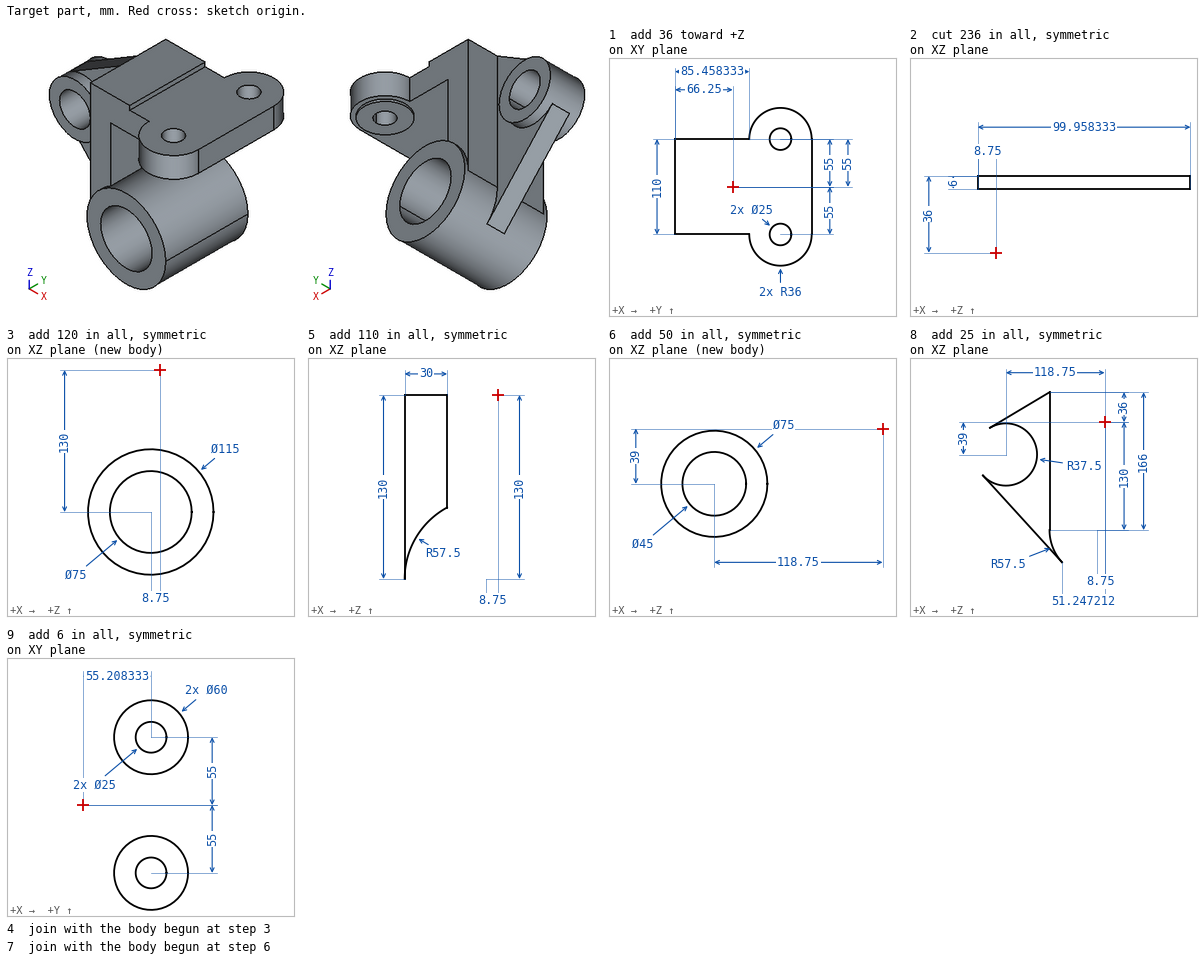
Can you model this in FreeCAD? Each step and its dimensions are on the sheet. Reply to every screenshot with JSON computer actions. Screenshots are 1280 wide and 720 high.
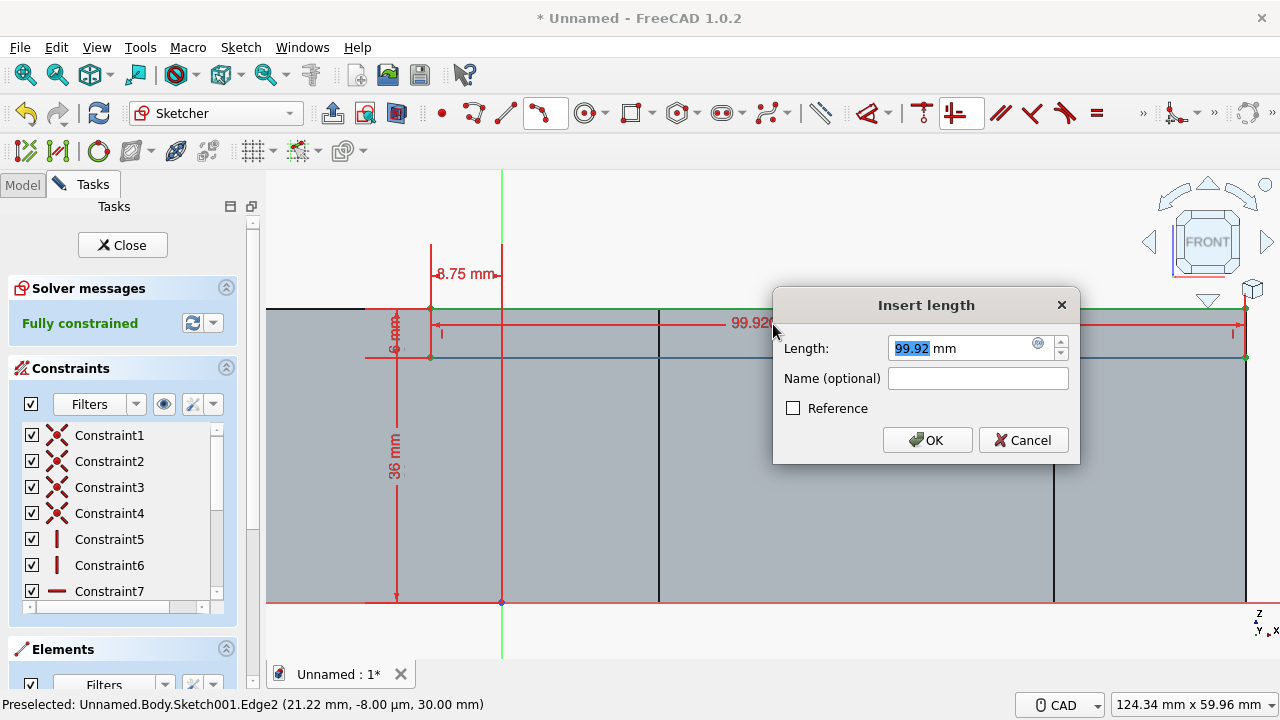
{"action": "type", "text": "99.958333"}
{"action": "key", "text": "Return"}
{"action": "key", "text": "Escape"}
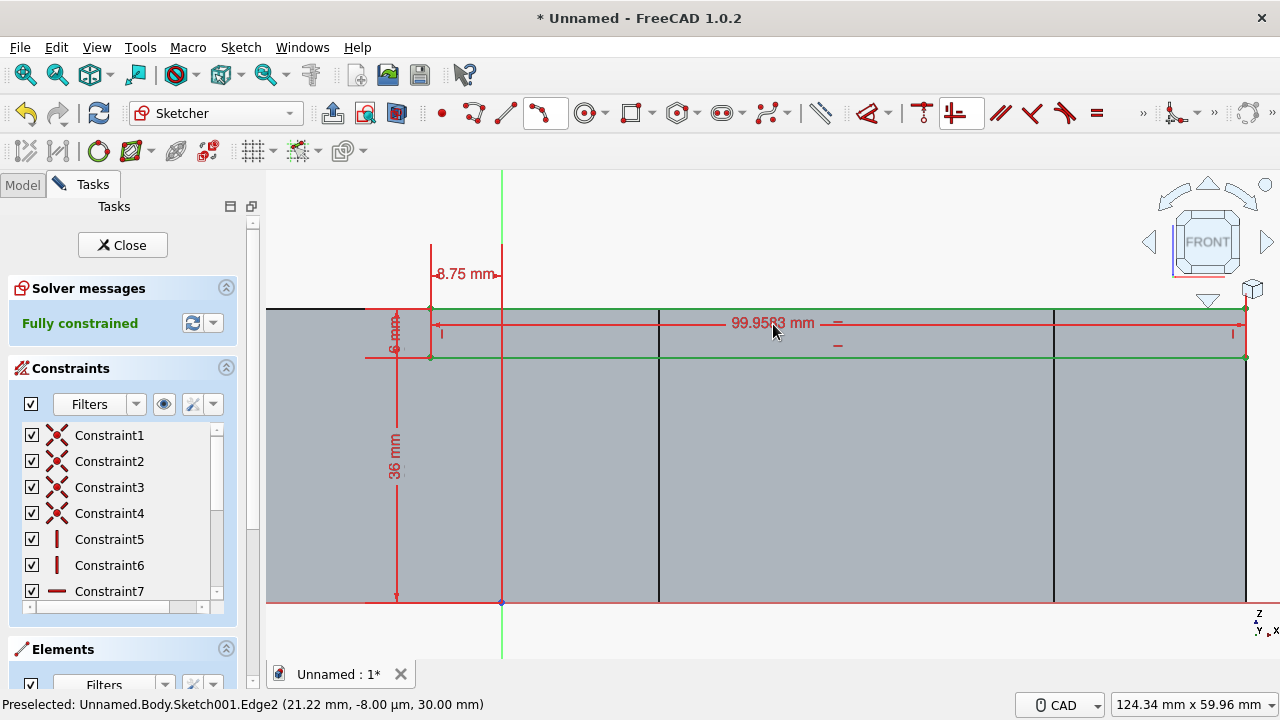
{"action": "left_click", "coordinate": [123, 245]}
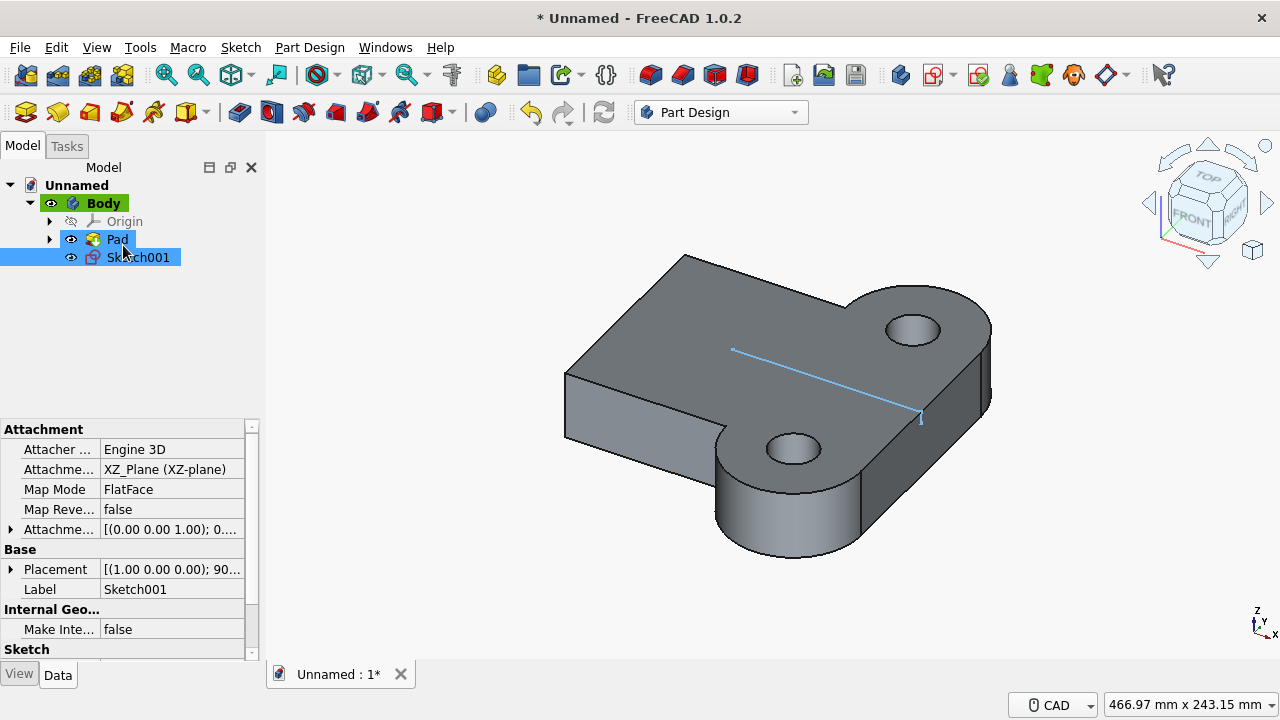
{"action": "left_click", "coordinate": [240, 112]}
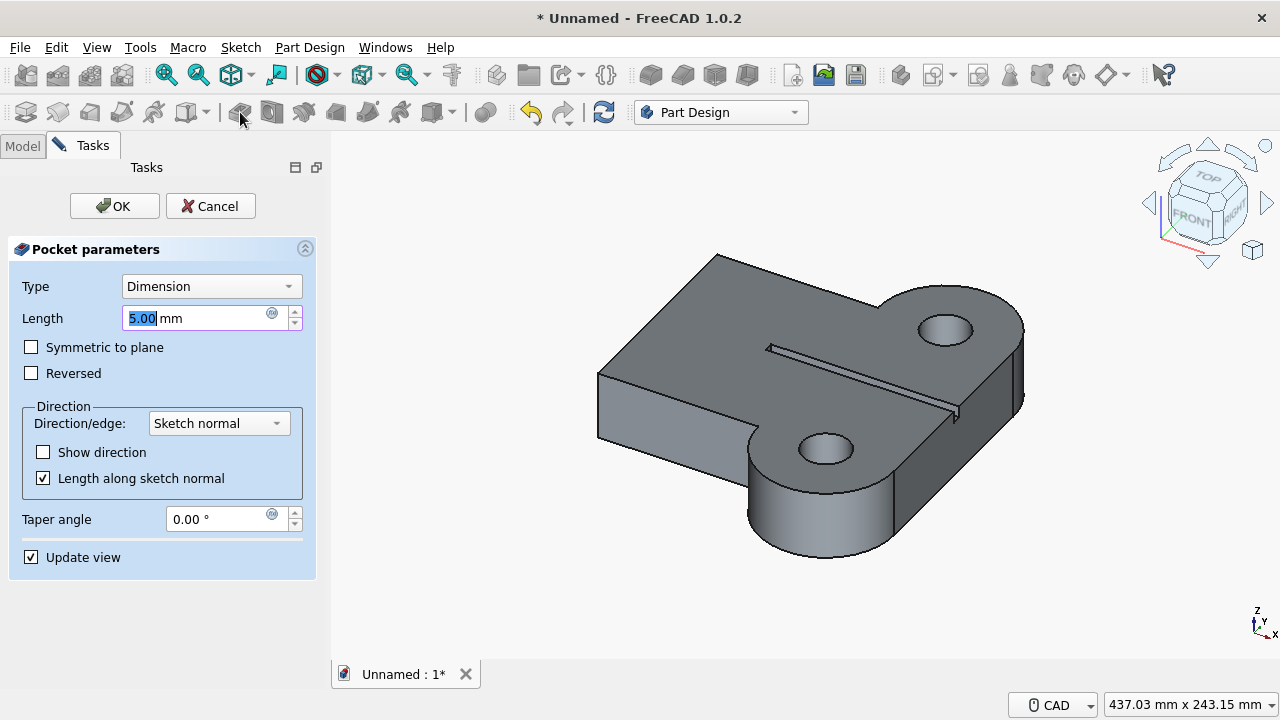
{"action": "type", "text": "236"}
{"action": "key", "text": "Tab"}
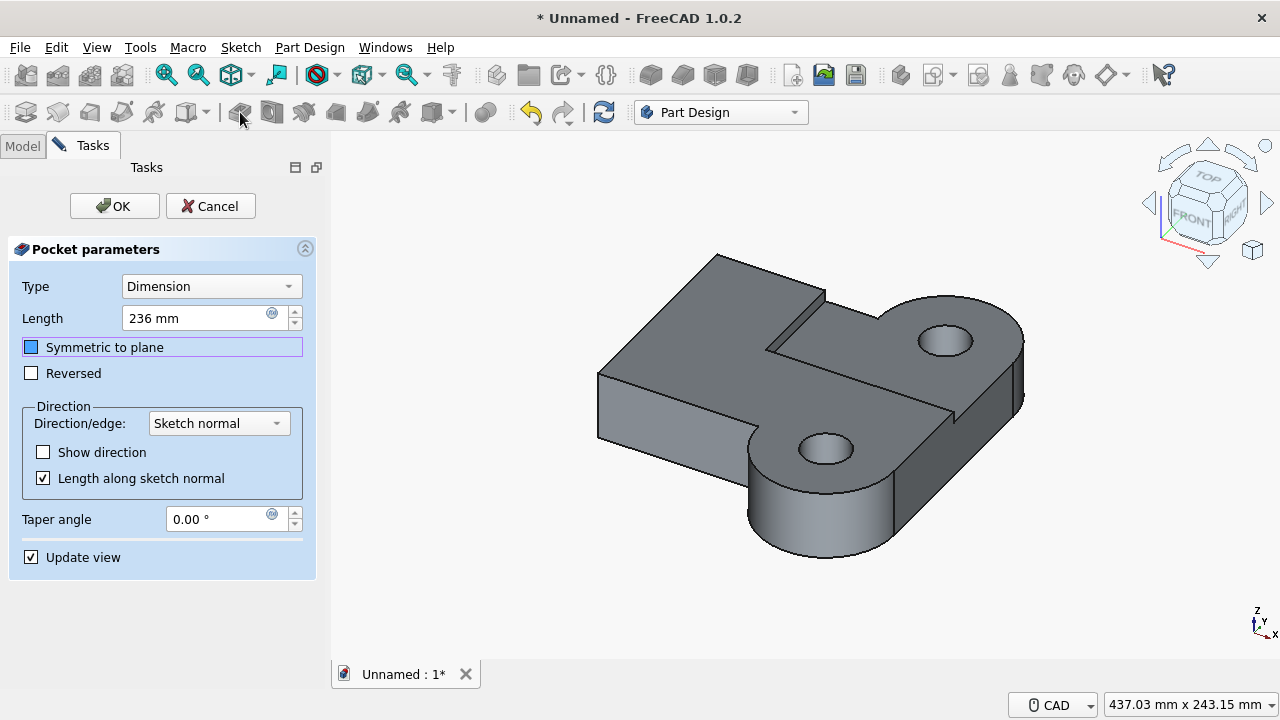
{"action": "left_click", "coordinate": [30, 347]}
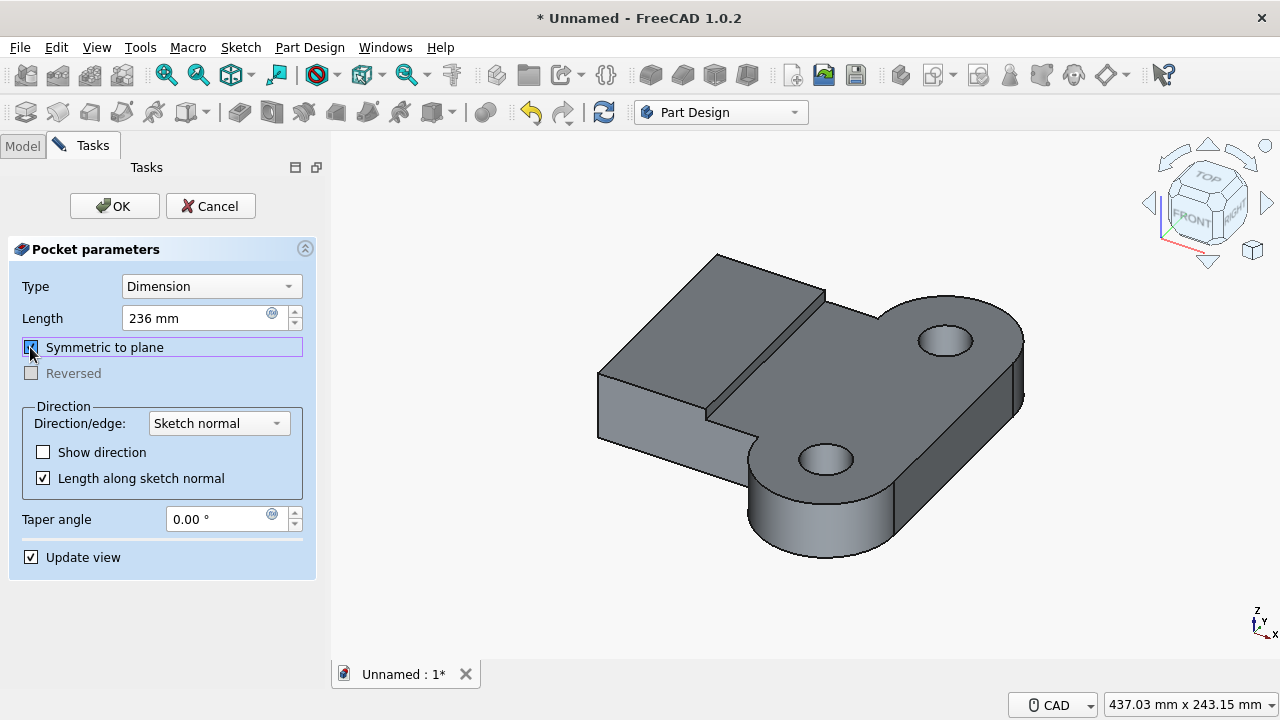
{"action": "left_click", "coordinate": [115, 206]}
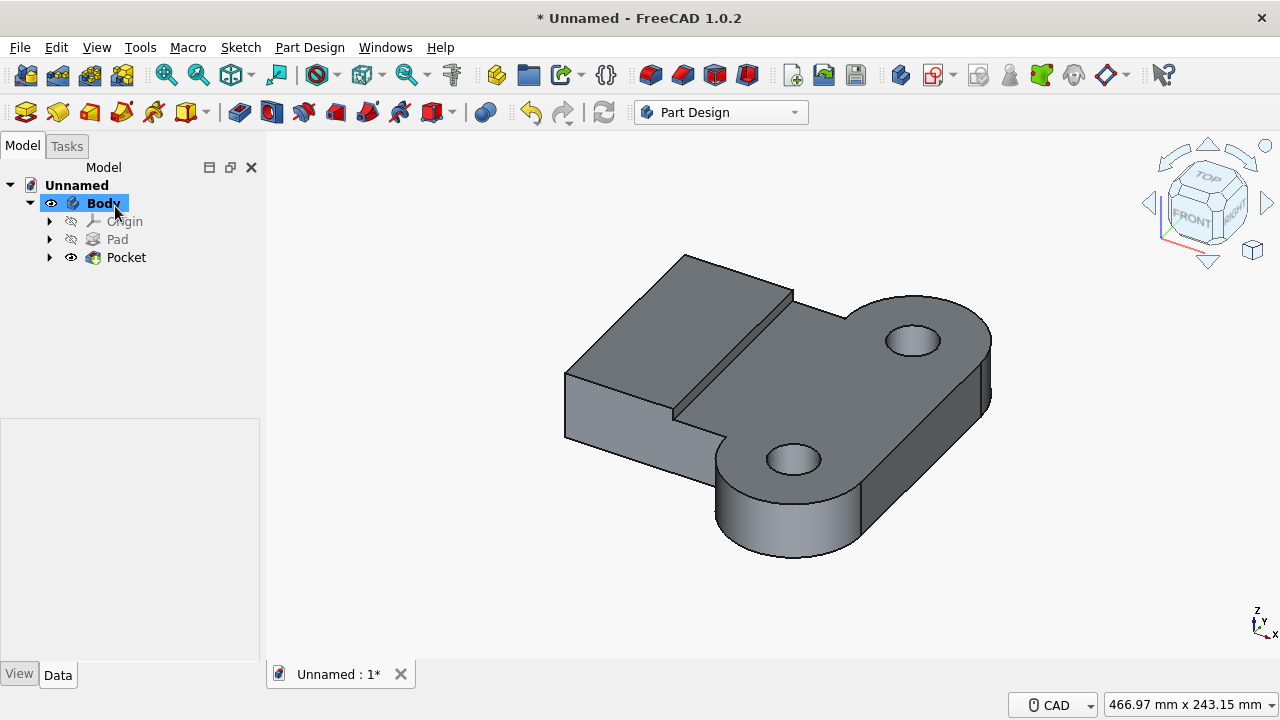
{"action": "left_click", "coordinate": [902, 76]}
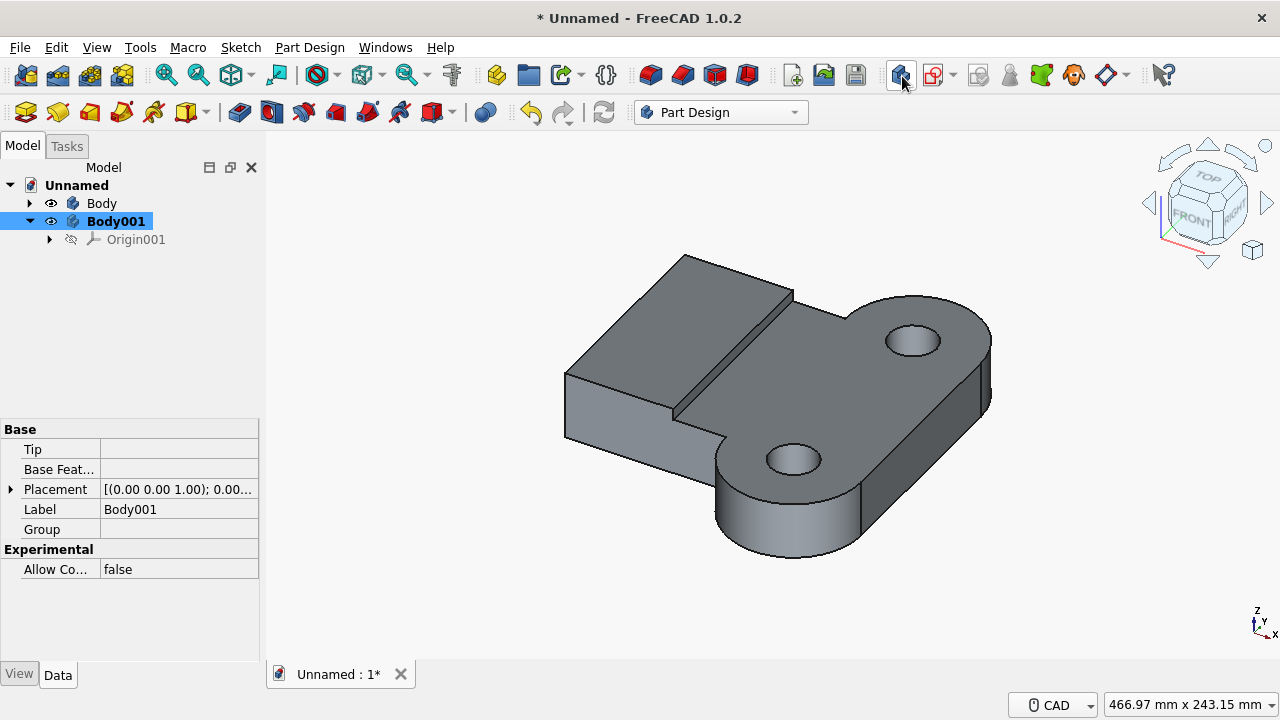
{"action": "left_click", "coordinate": [306, 619]}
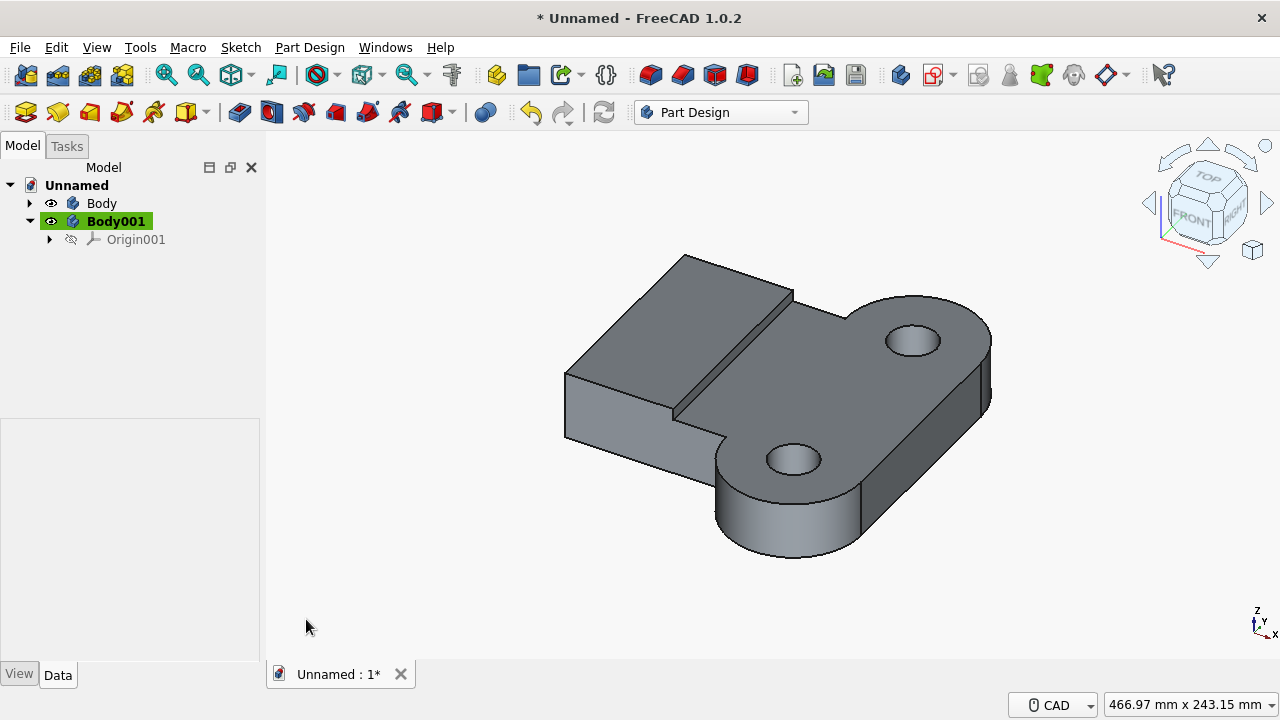
{"action": "left_click", "coordinate": [934, 76]}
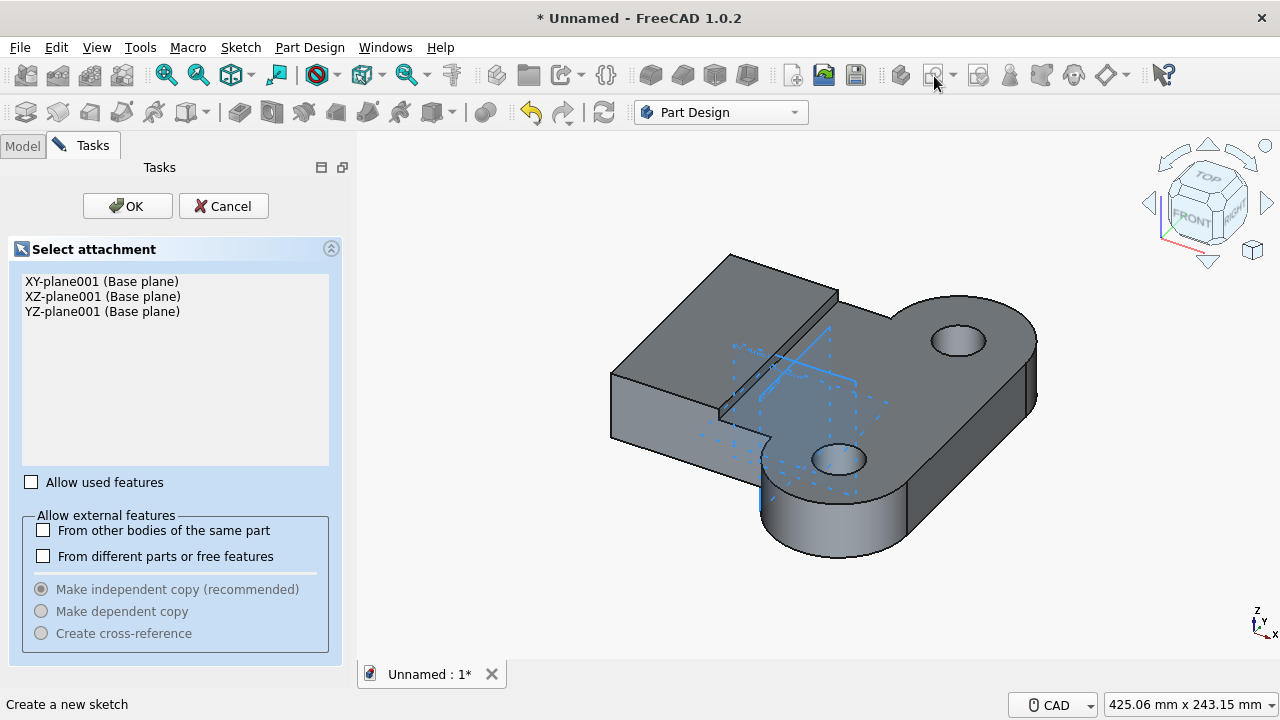
{"action": "left_click", "coordinate": [82, 296]}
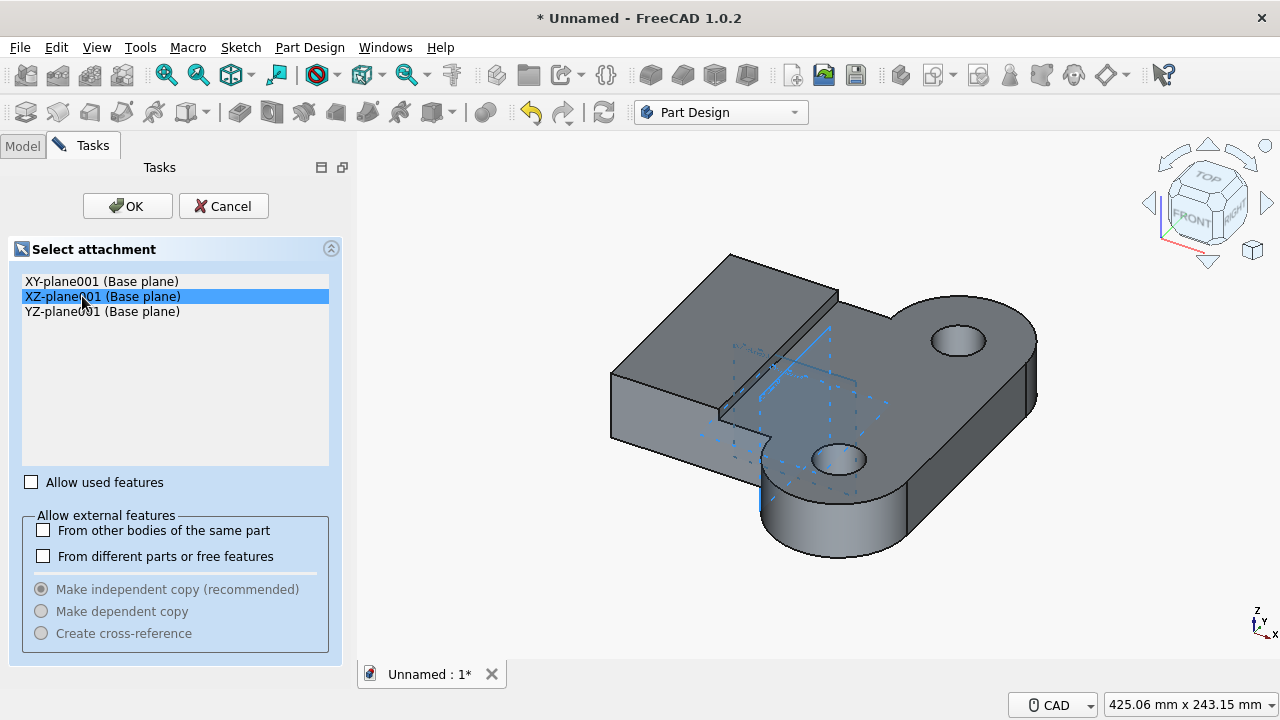
{"action": "left_click", "coordinate": [128, 206]}